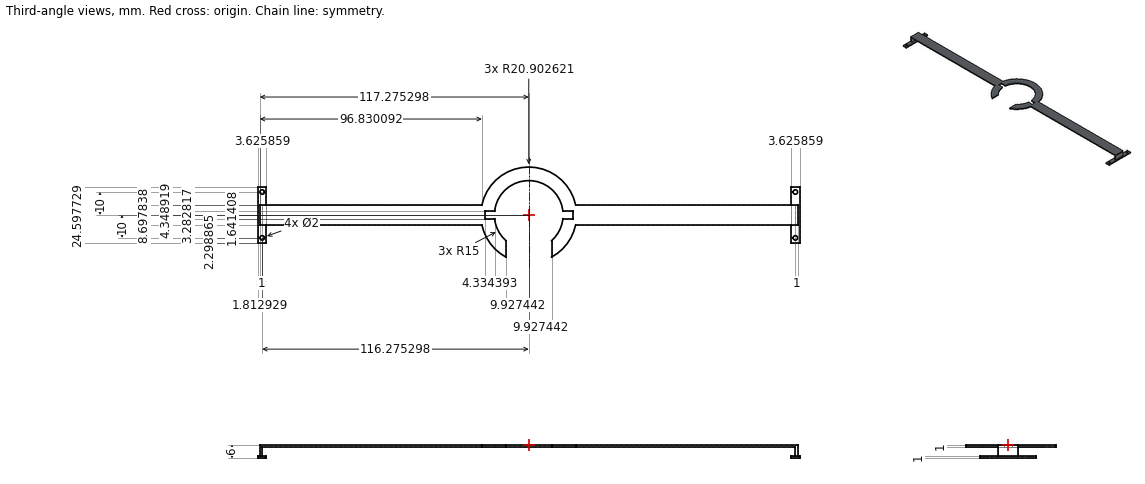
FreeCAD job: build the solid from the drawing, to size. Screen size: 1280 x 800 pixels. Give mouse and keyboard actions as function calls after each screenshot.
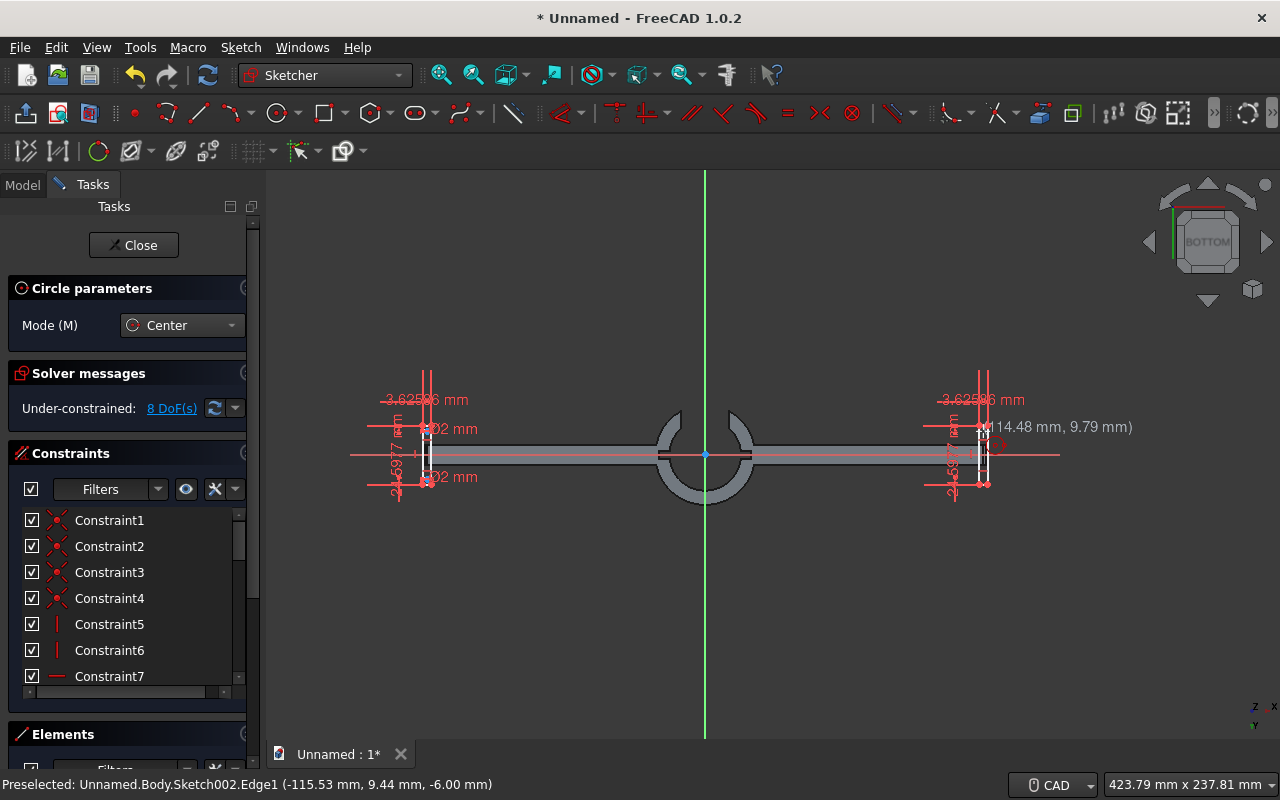
scroll(983, 431, up, 7)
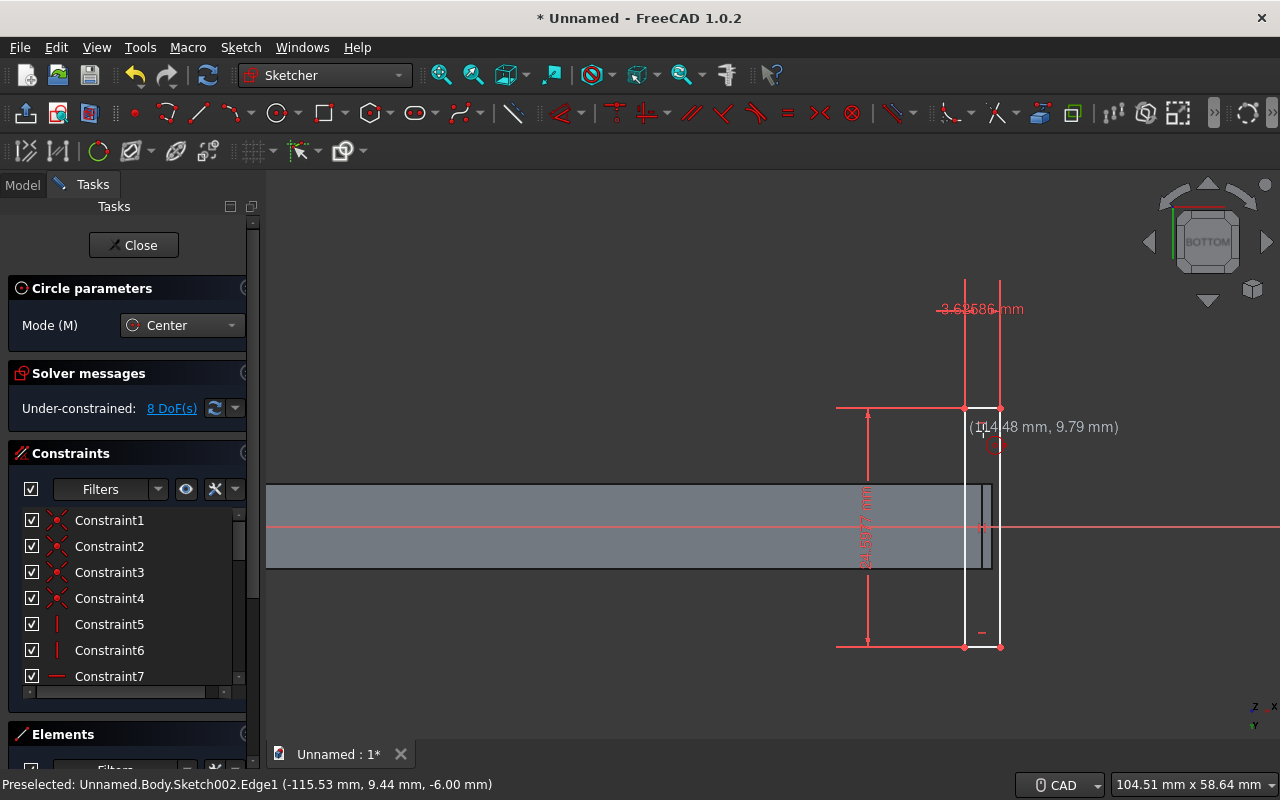
click(982, 430)
move(979, 439)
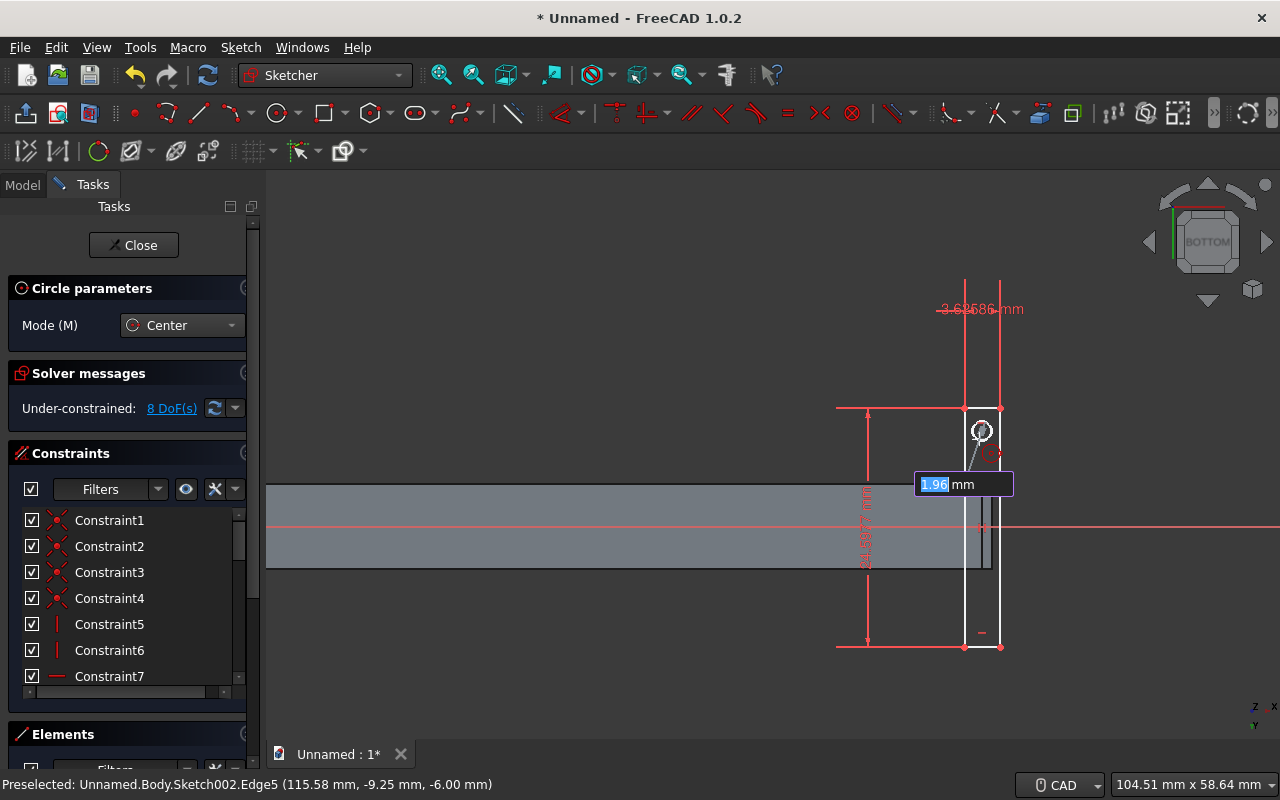
text(2)
key(Return)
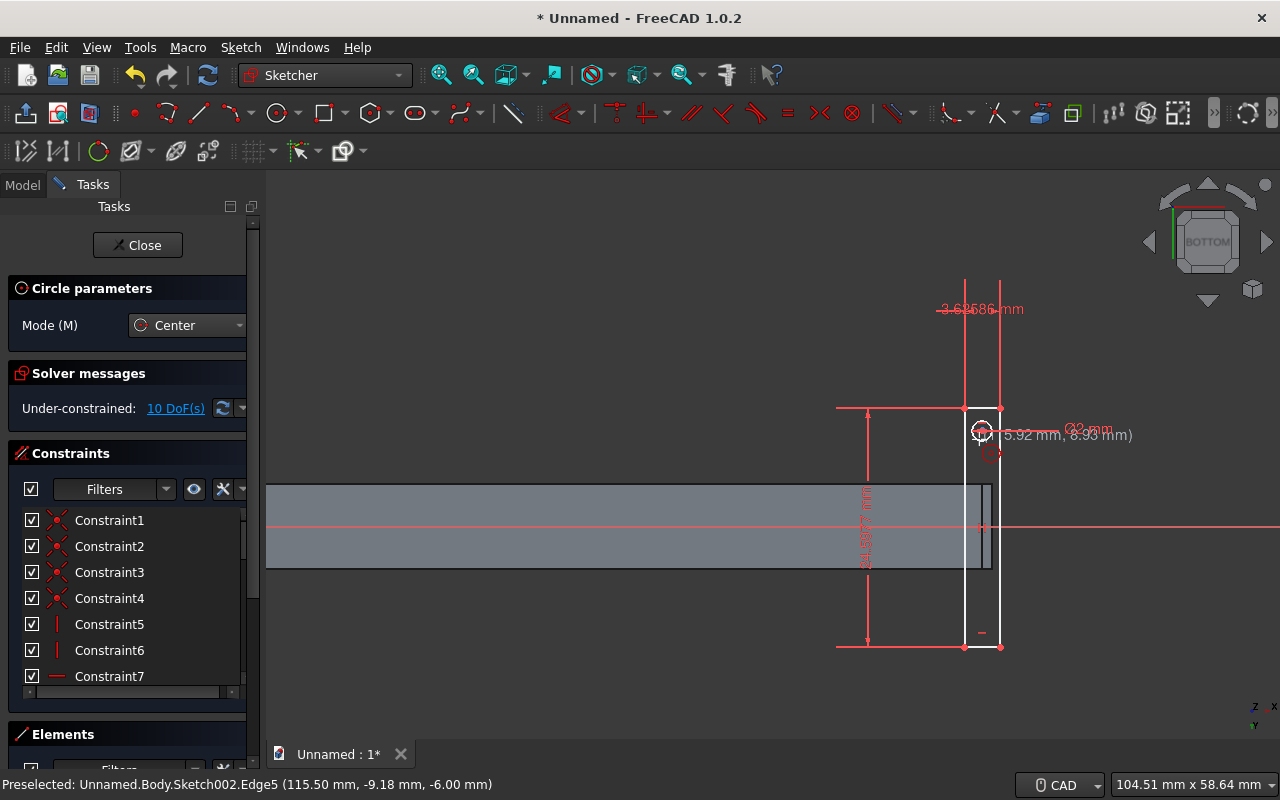
scroll(982, 624, up, 5)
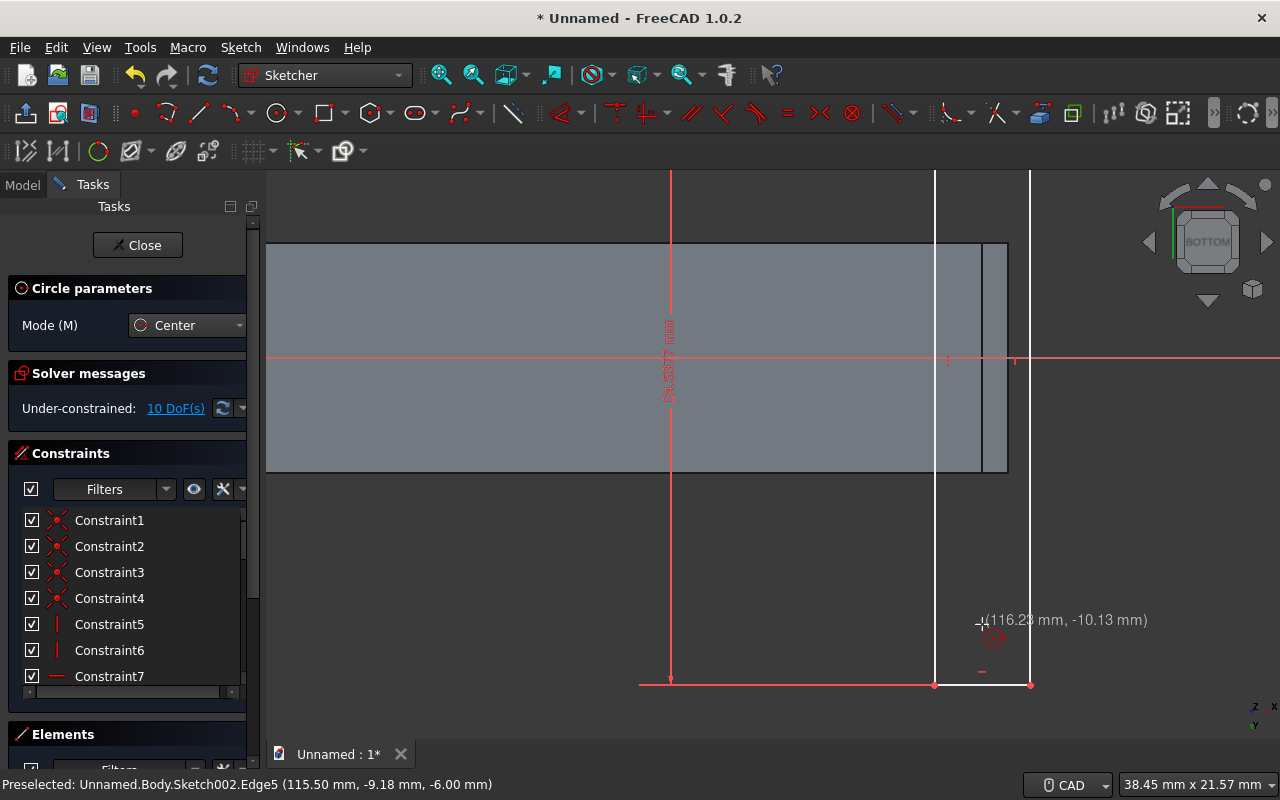
scroll(983, 464, down, 12)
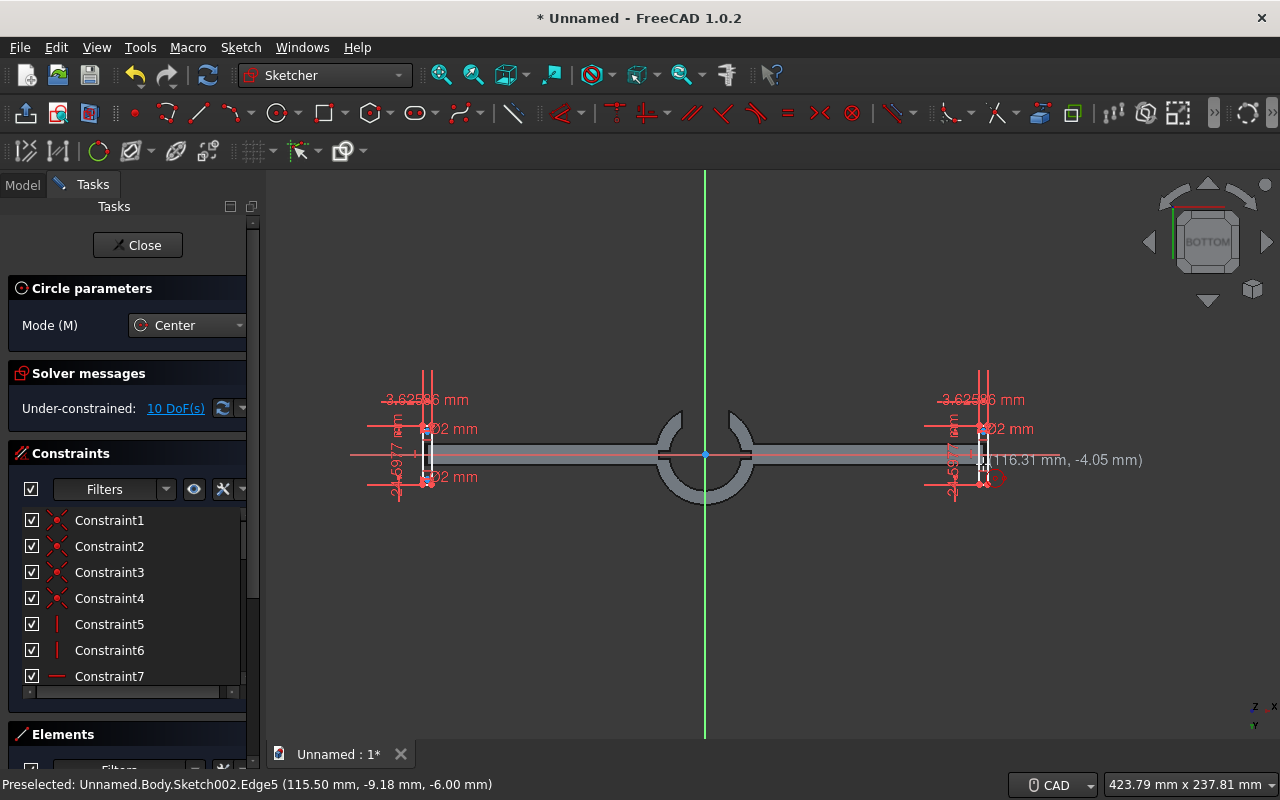
scroll(984, 479, up, 7)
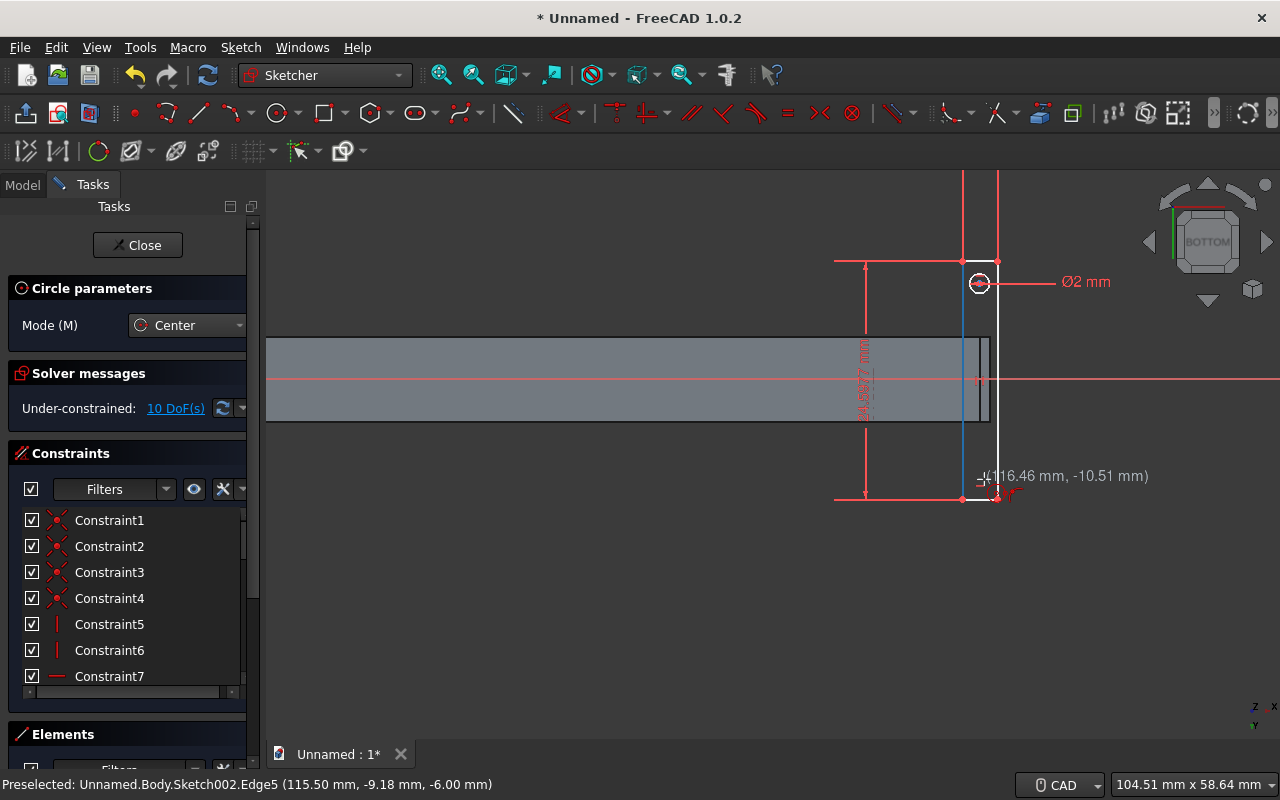
click(980, 476)
move(983, 467)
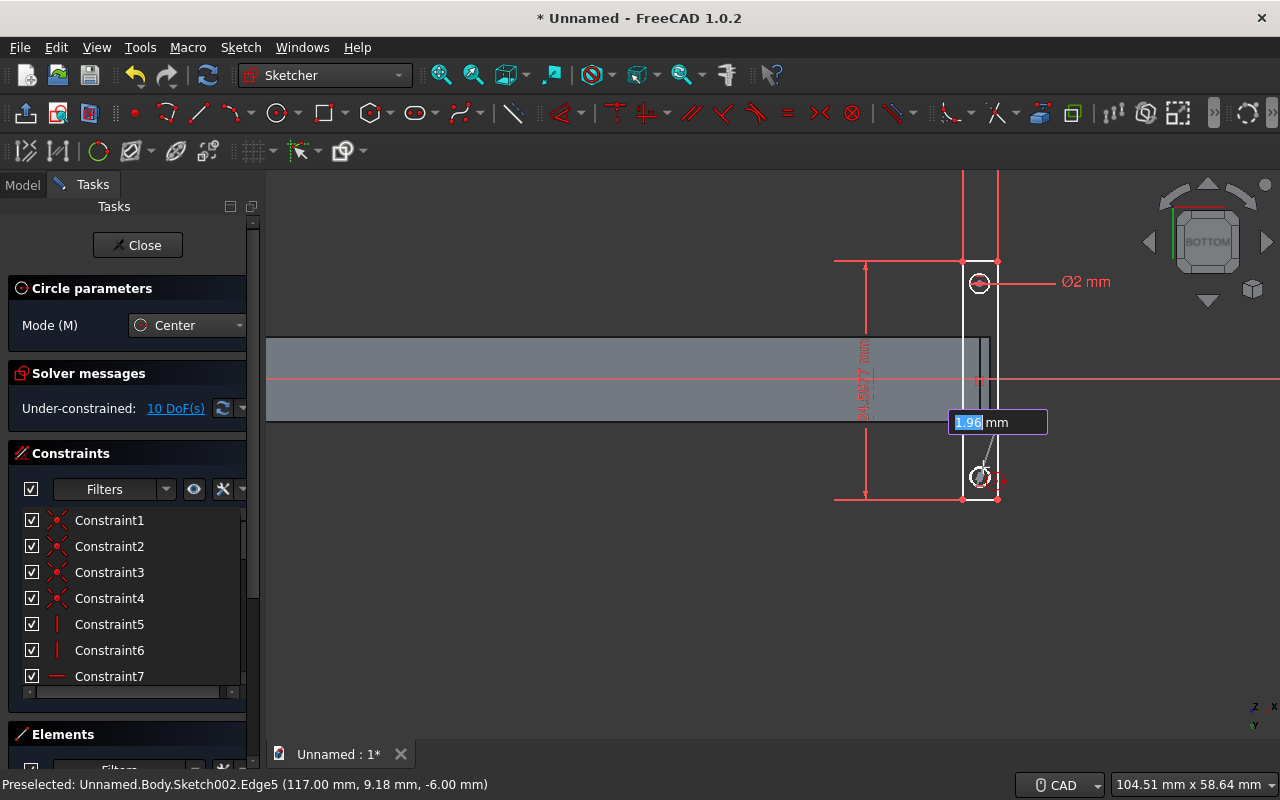
text(2)
key(Return)
key(Escape)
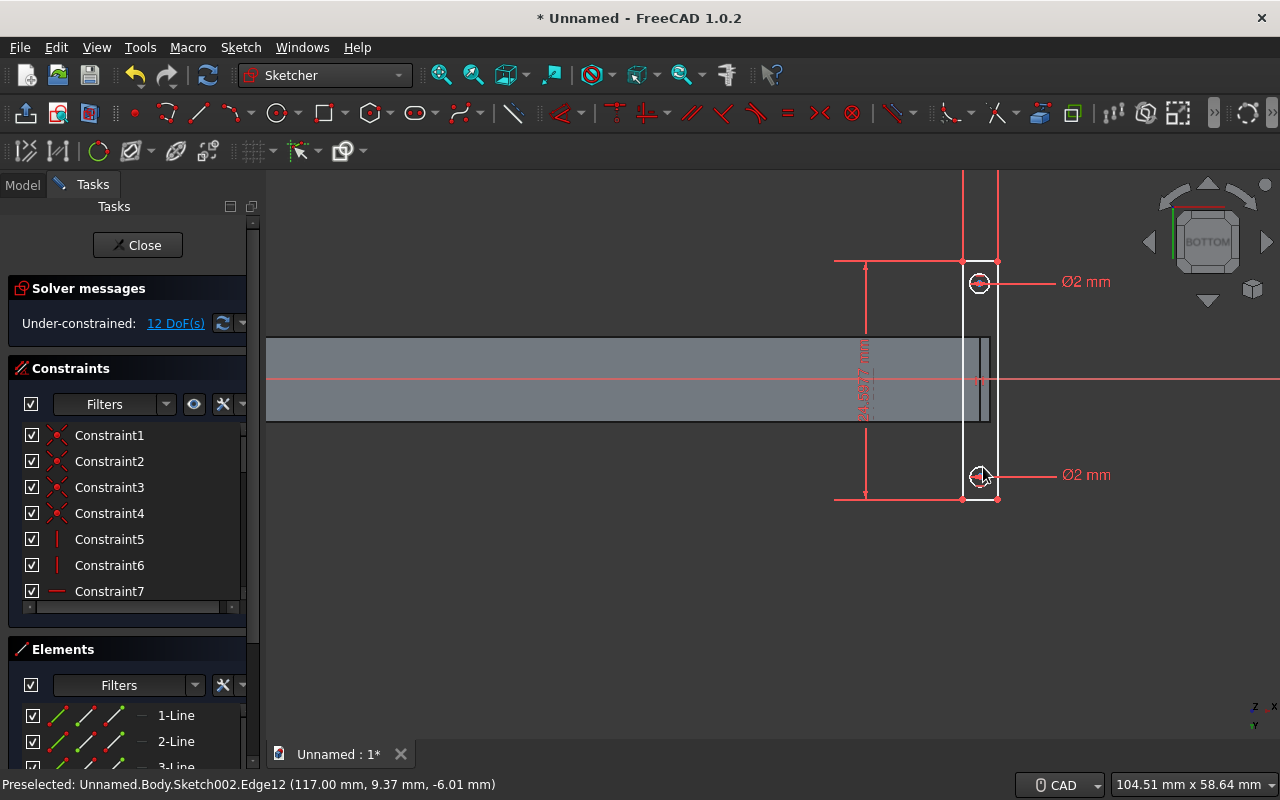
scroll(984, 479, down, 7)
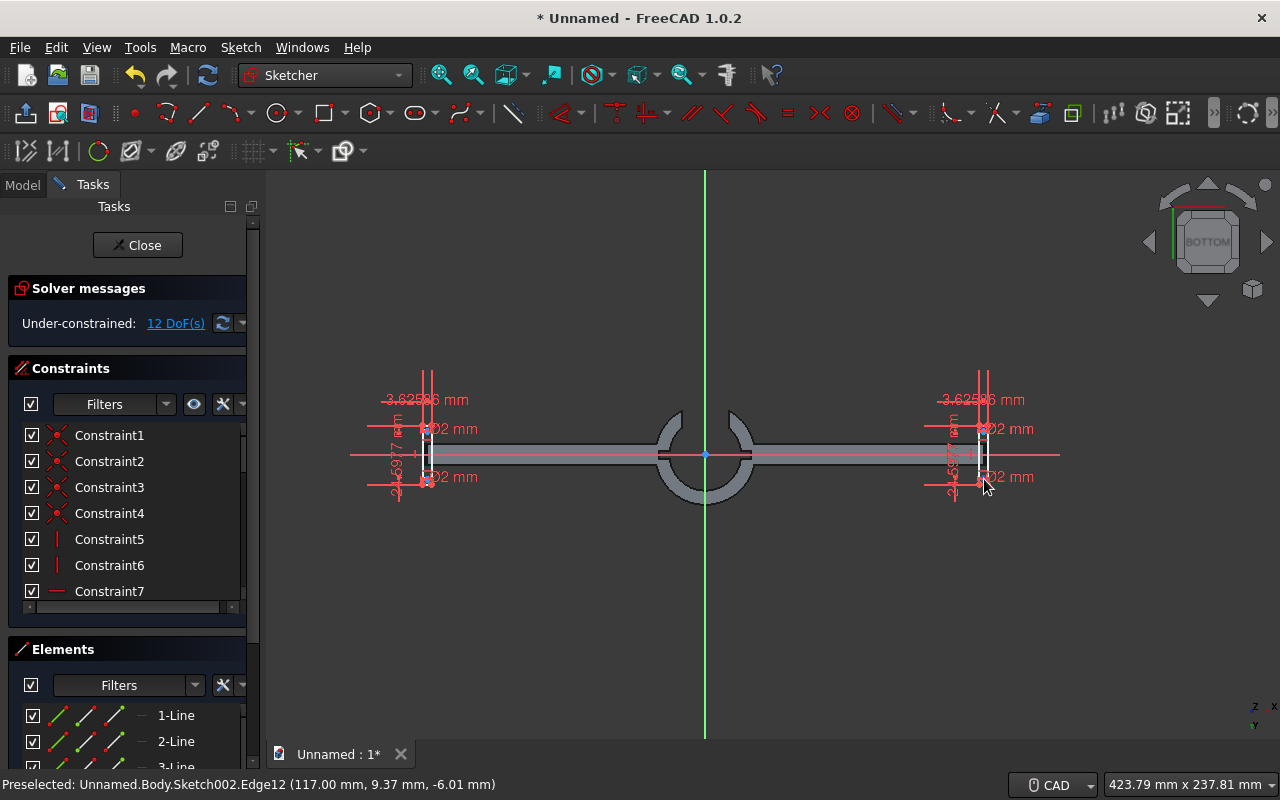
scroll(427, 431, up, 3)